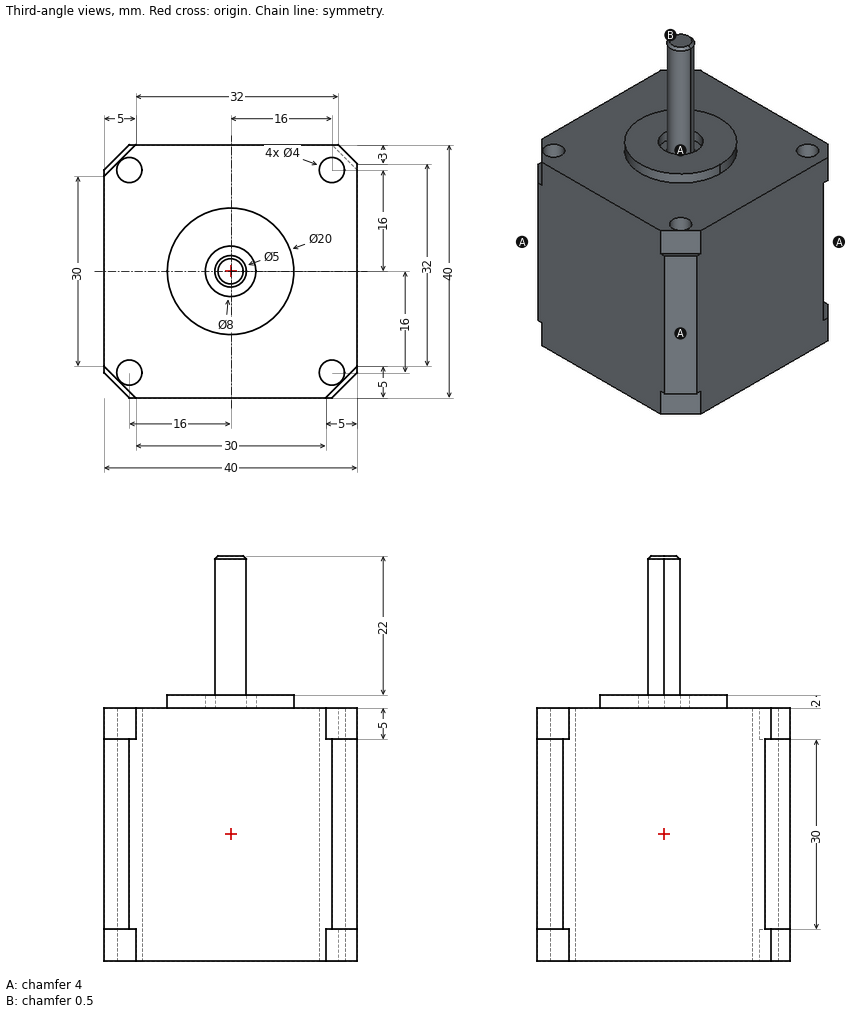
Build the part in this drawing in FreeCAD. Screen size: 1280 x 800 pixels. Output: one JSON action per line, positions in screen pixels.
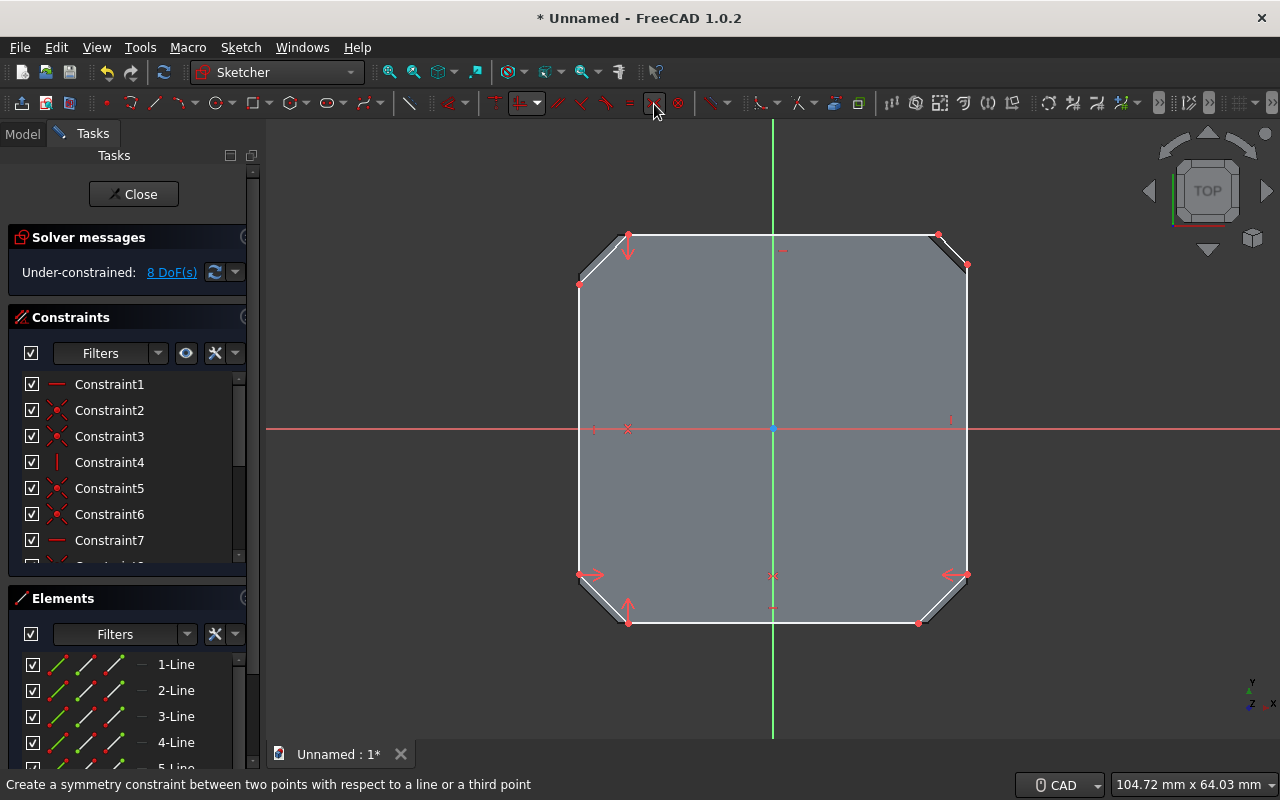
{"action": "left_click", "coordinate": [715, 623]}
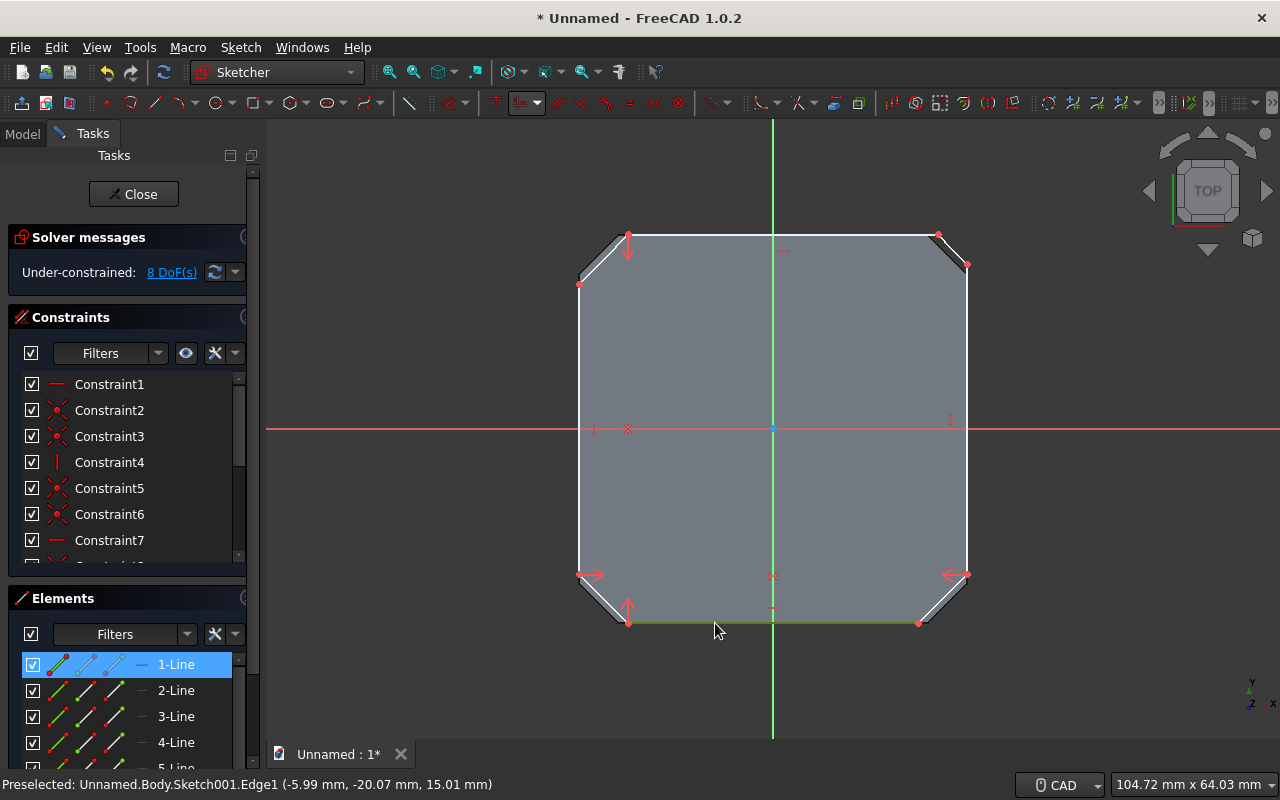
{"action": "left_click", "coordinate": [468, 104]}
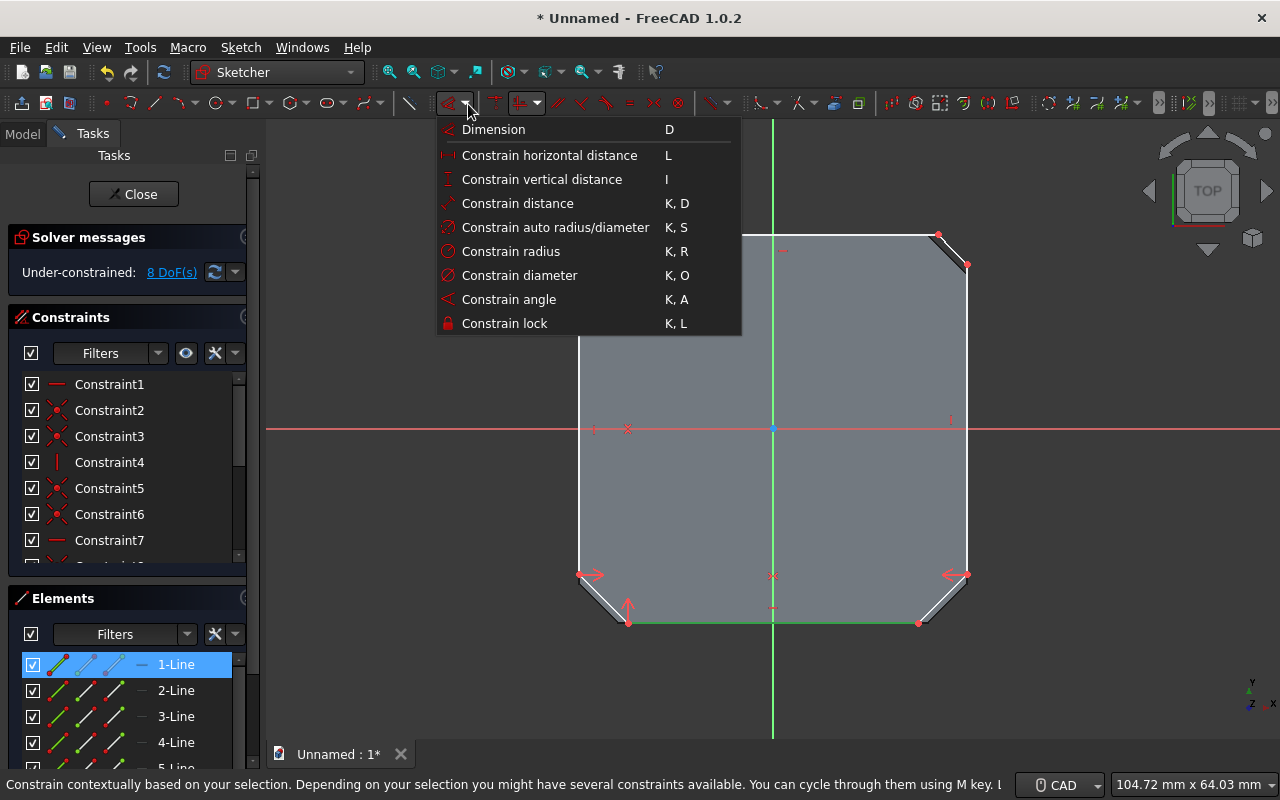
{"action": "left_click", "coordinate": [589, 155]}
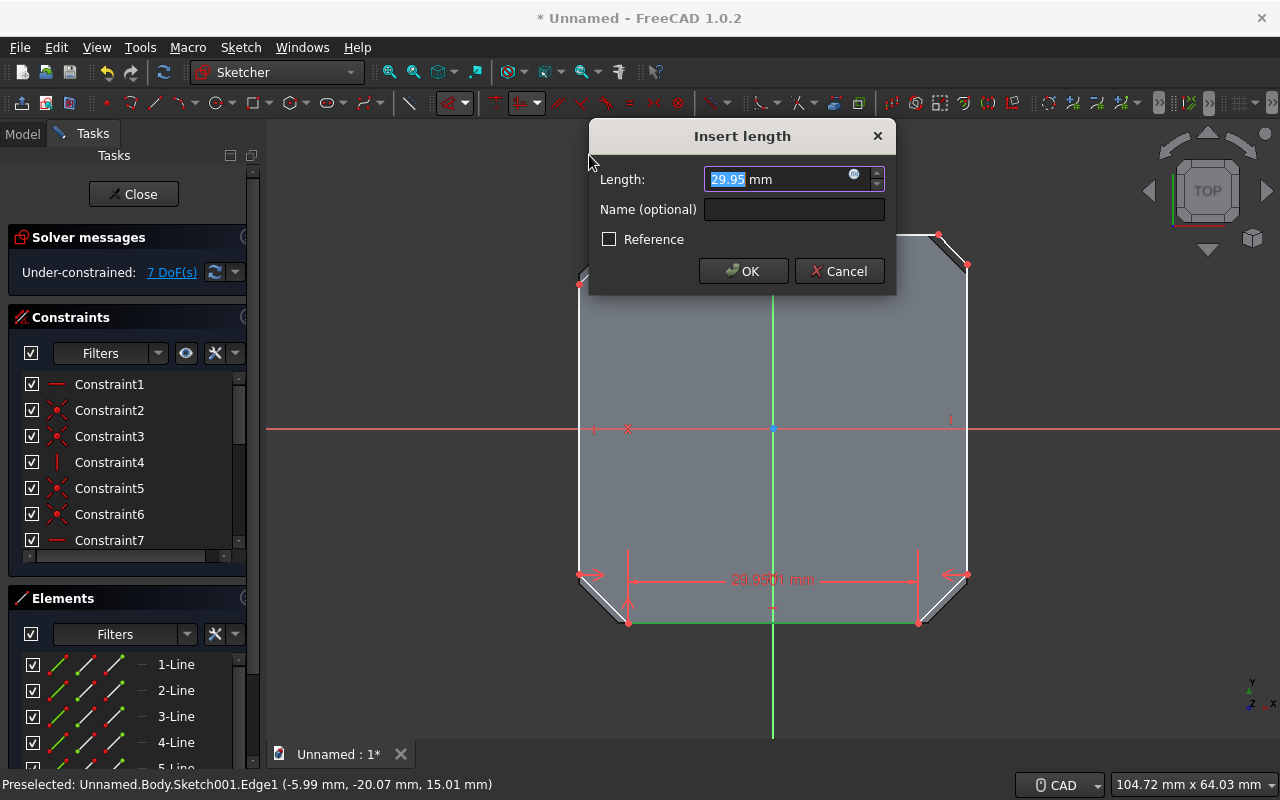
{"action": "type", "text": "30"}
{"action": "key", "text": "Return"}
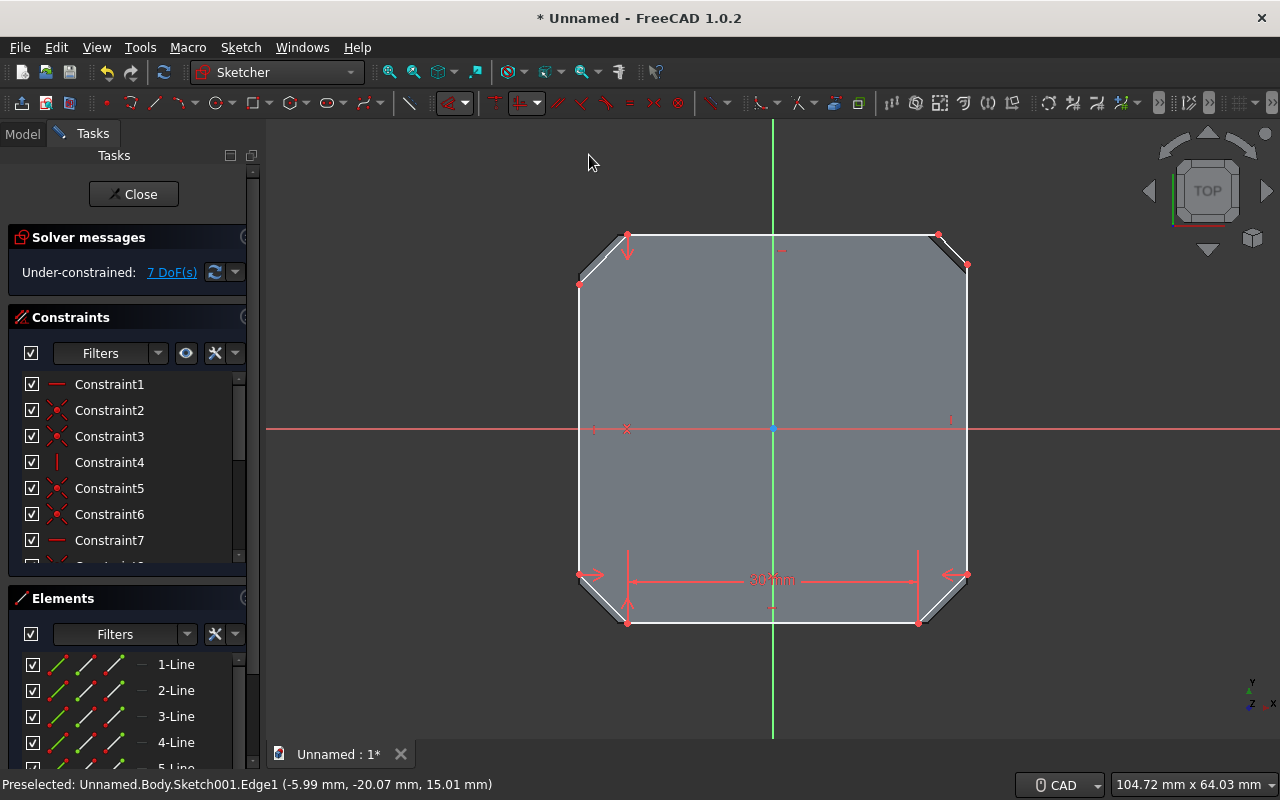
{"action": "left_click", "coordinate": [967, 482]}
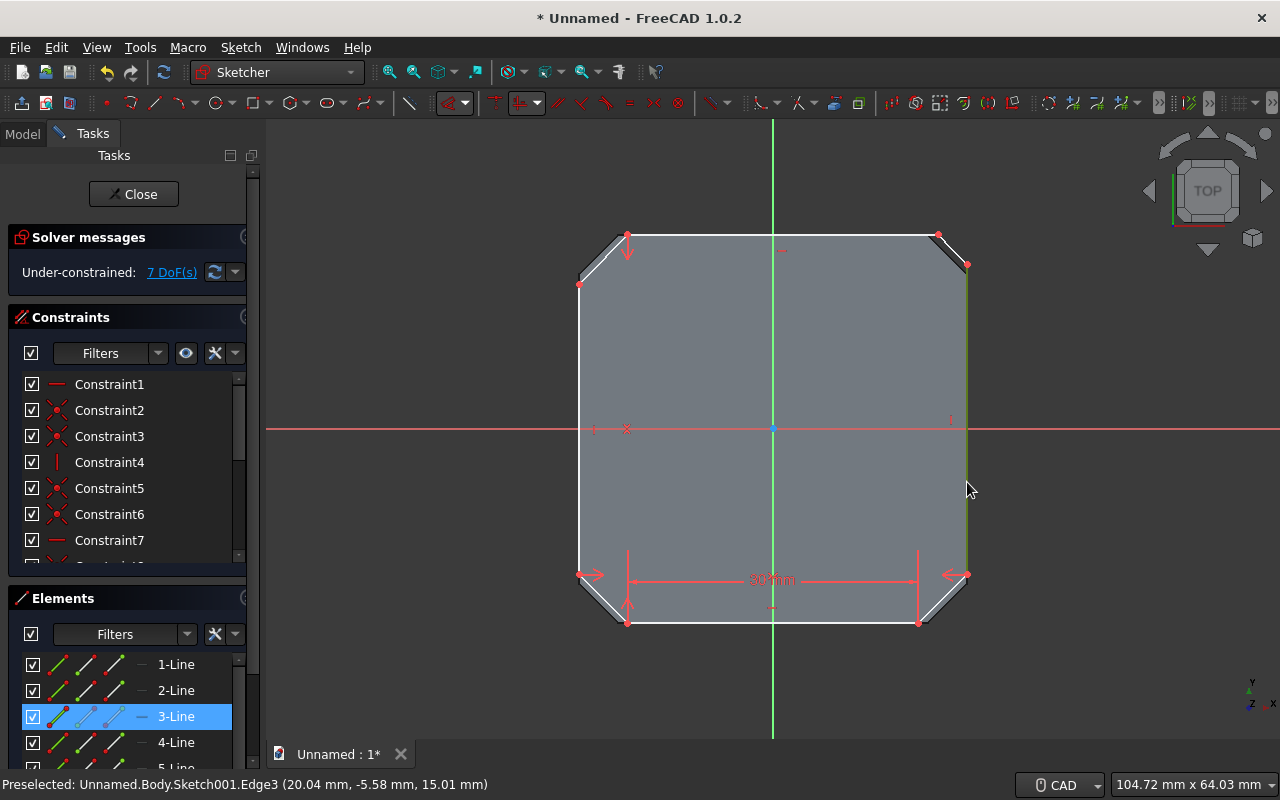
{"action": "left_click", "coordinate": [468, 104]}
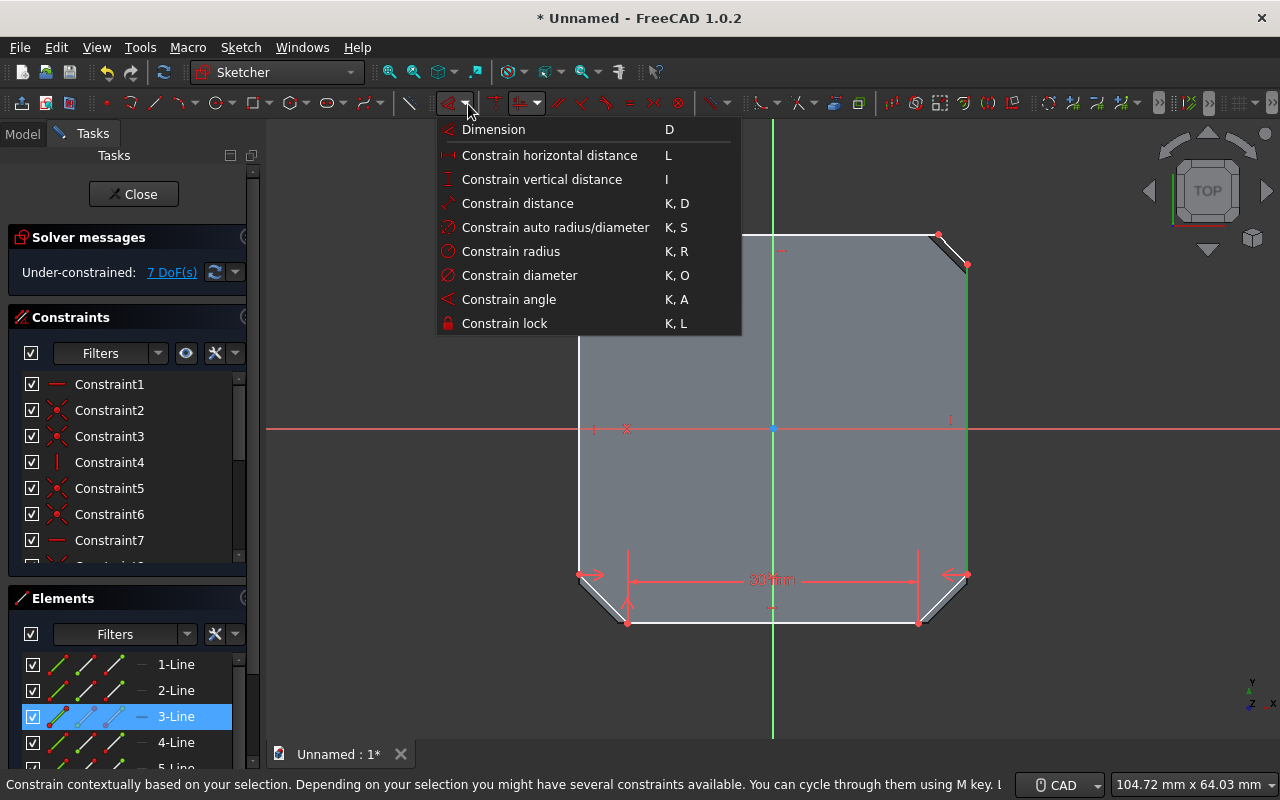
{"action": "left_click", "coordinate": [589, 179]}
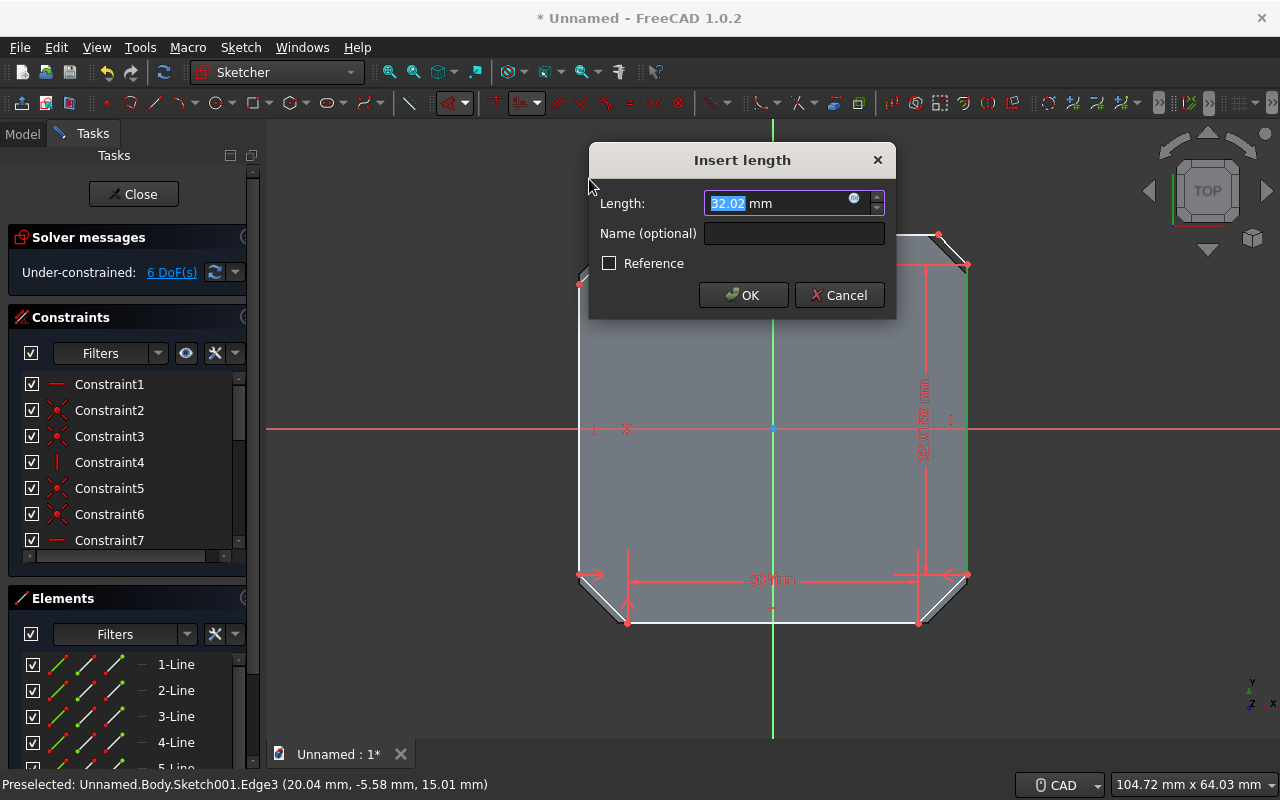
{"action": "type", "text": "32"}
{"action": "key", "text": "Return"}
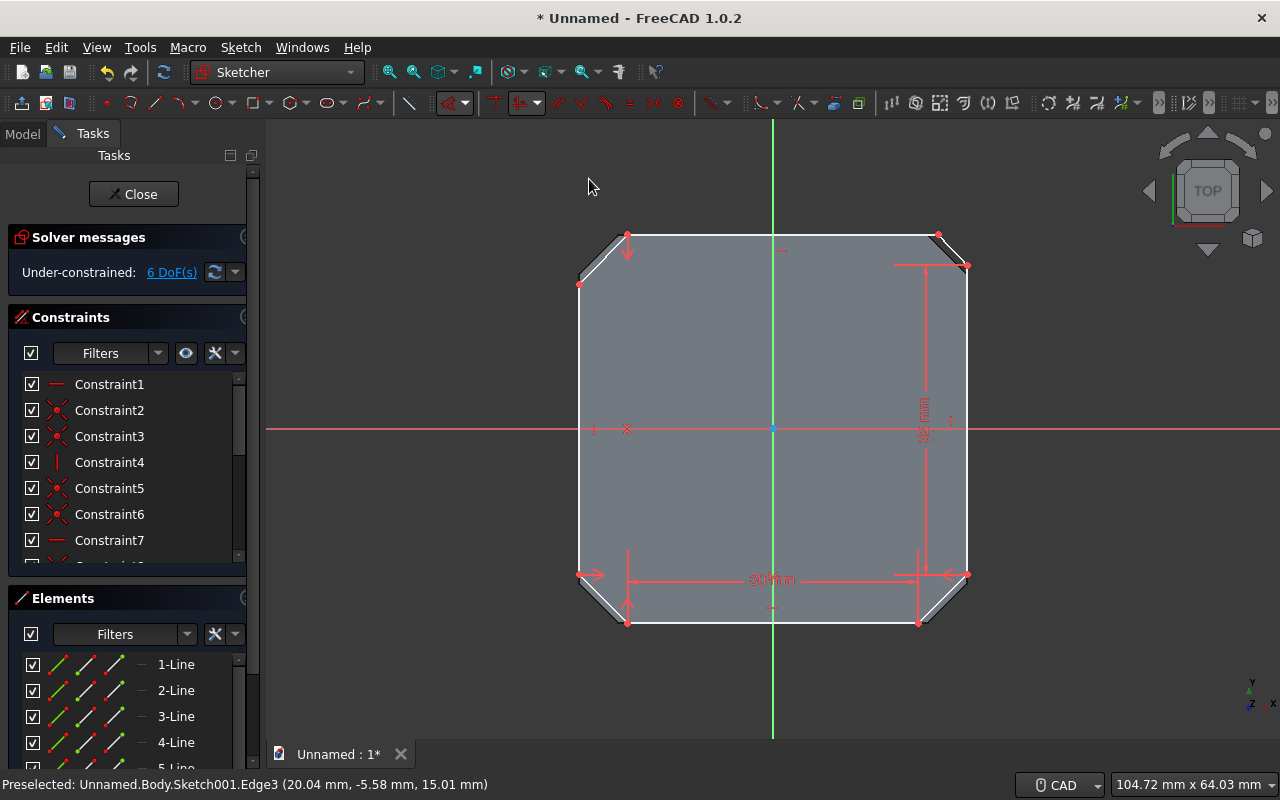
{"action": "left_click", "coordinate": [845, 235]}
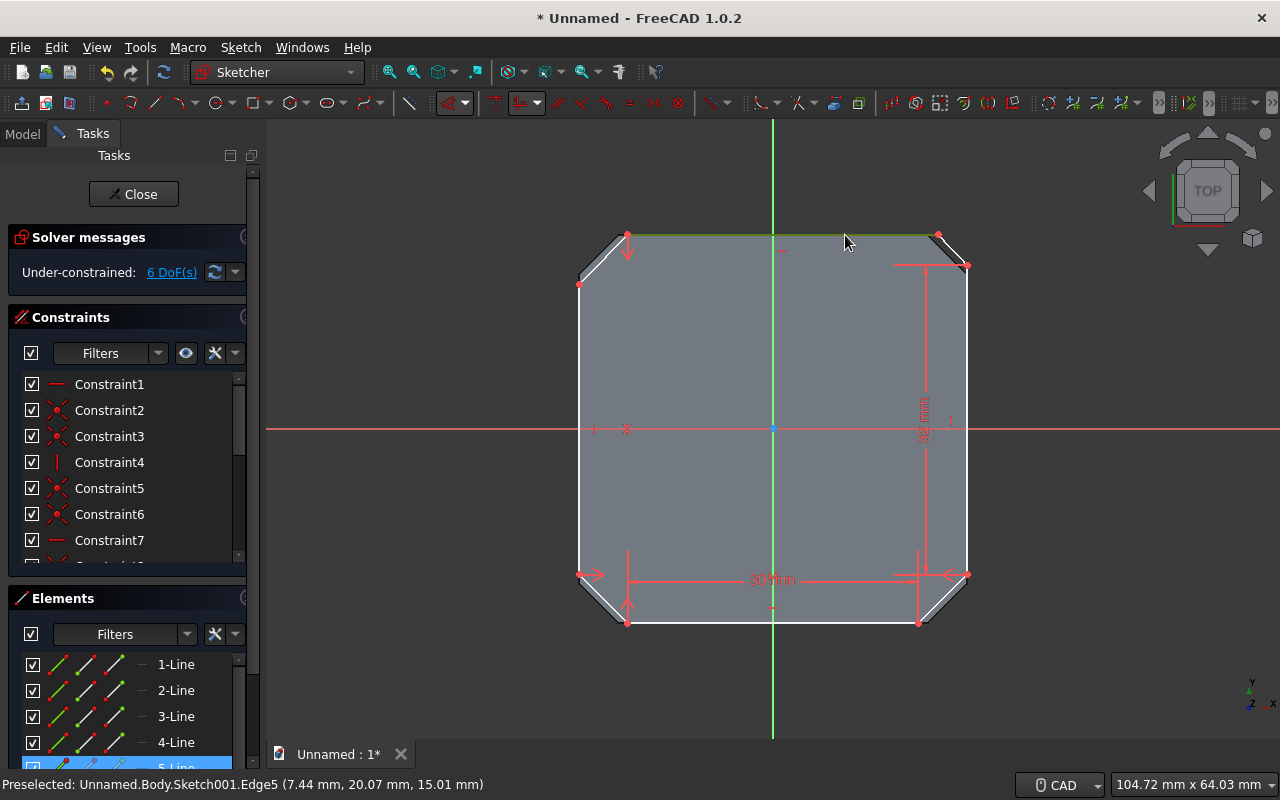
{"action": "left_click", "coordinate": [468, 104]}